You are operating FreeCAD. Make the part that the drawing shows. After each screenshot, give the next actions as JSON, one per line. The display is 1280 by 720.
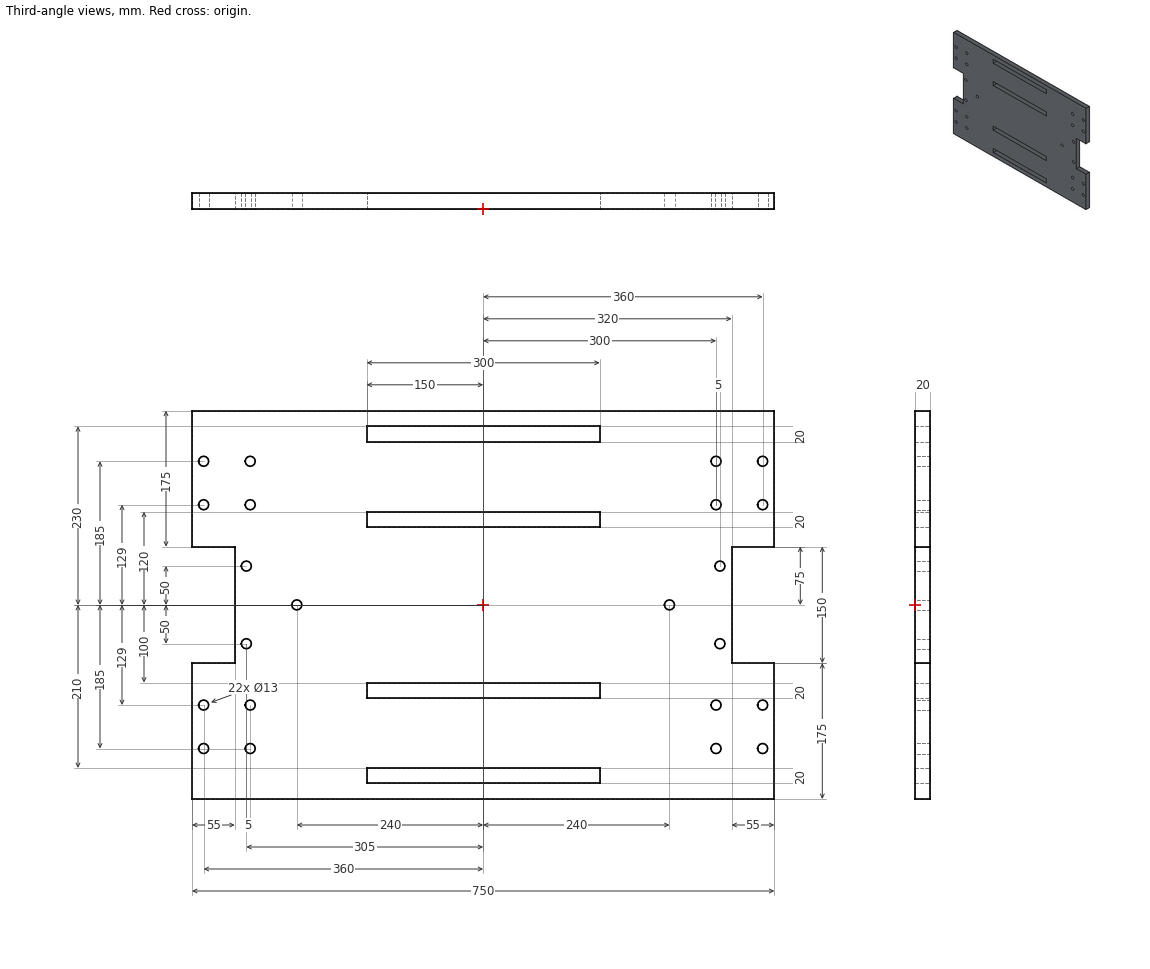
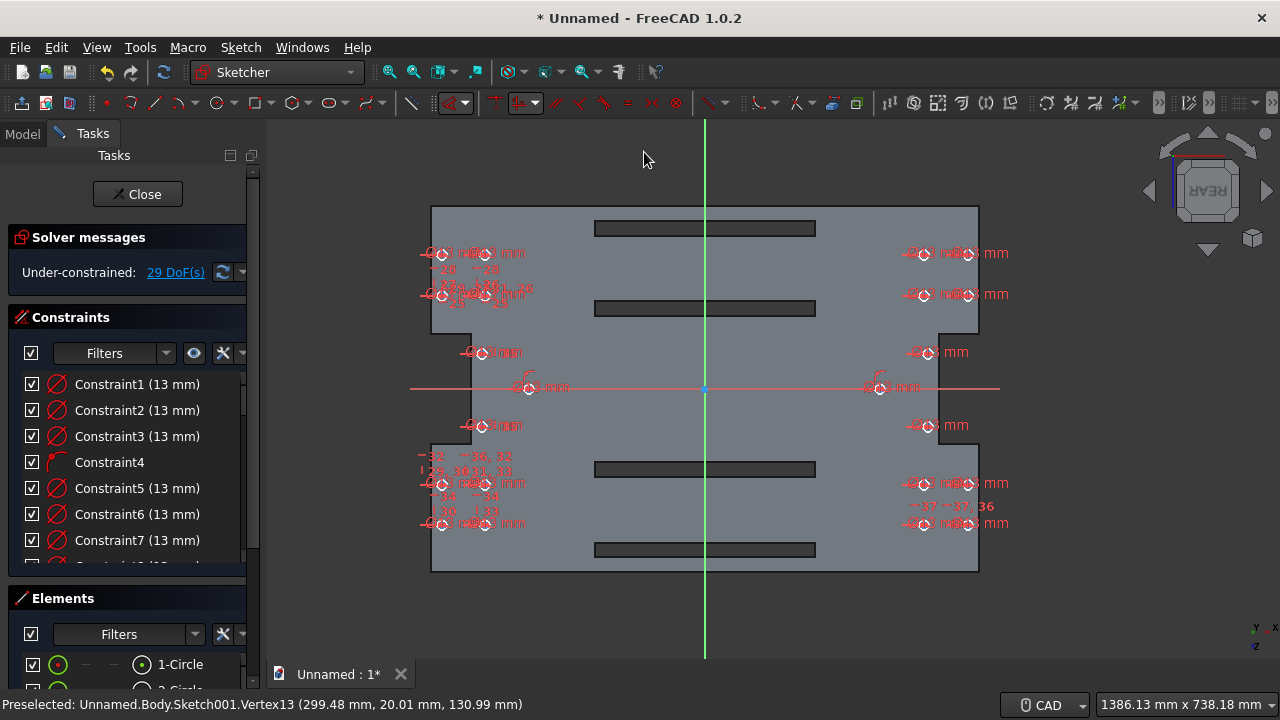
{"action": "left_click", "coordinate": [968, 485]}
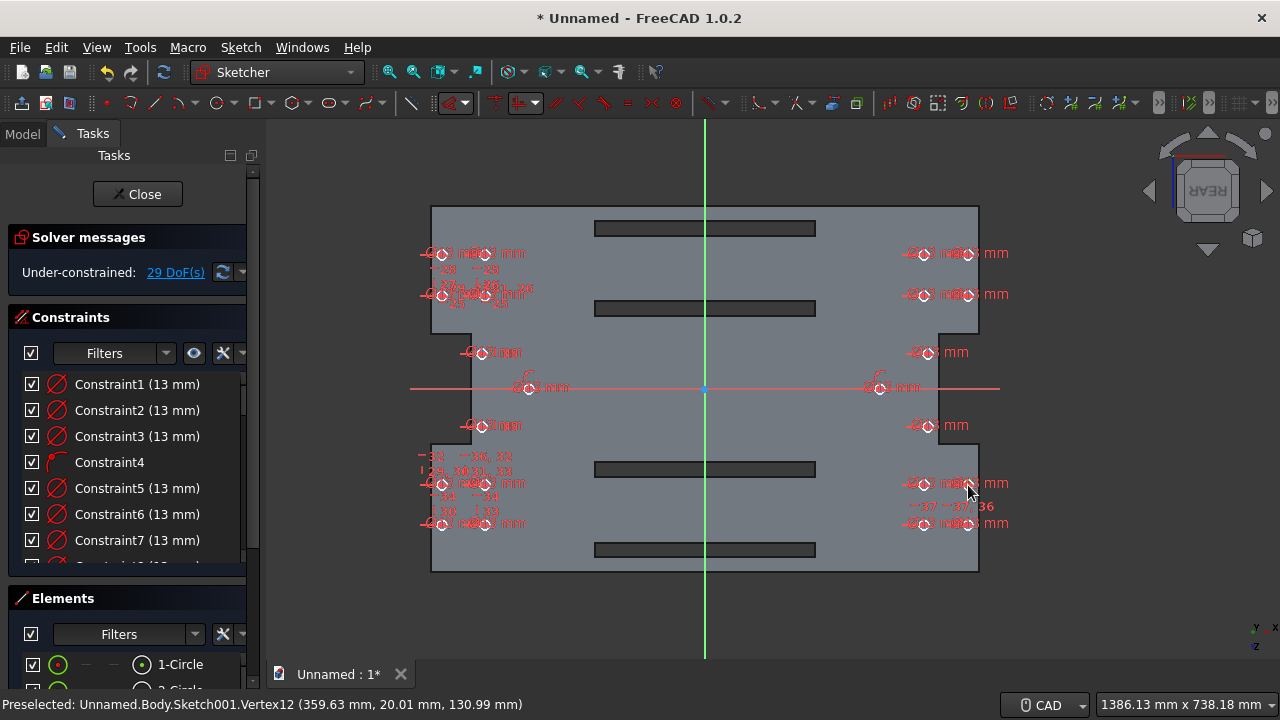
{"action": "left_click", "coordinate": [968, 525]}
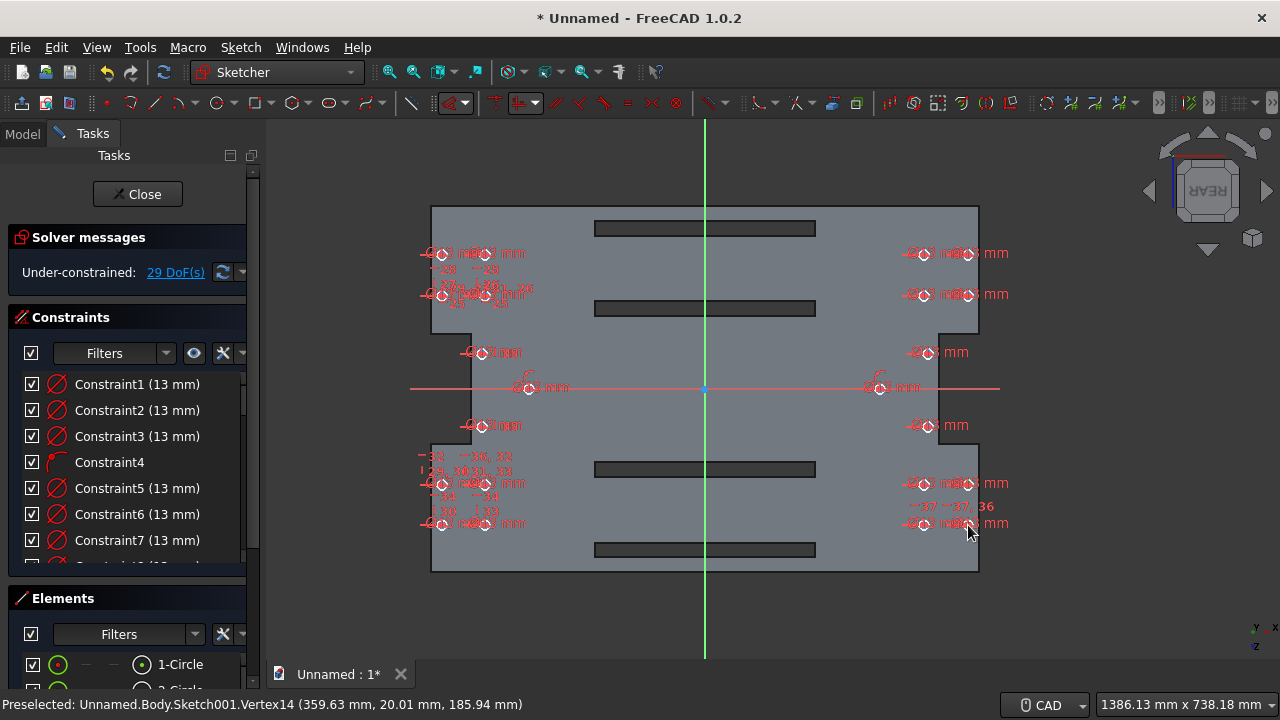
{"action": "left_click", "coordinate": [538, 104]}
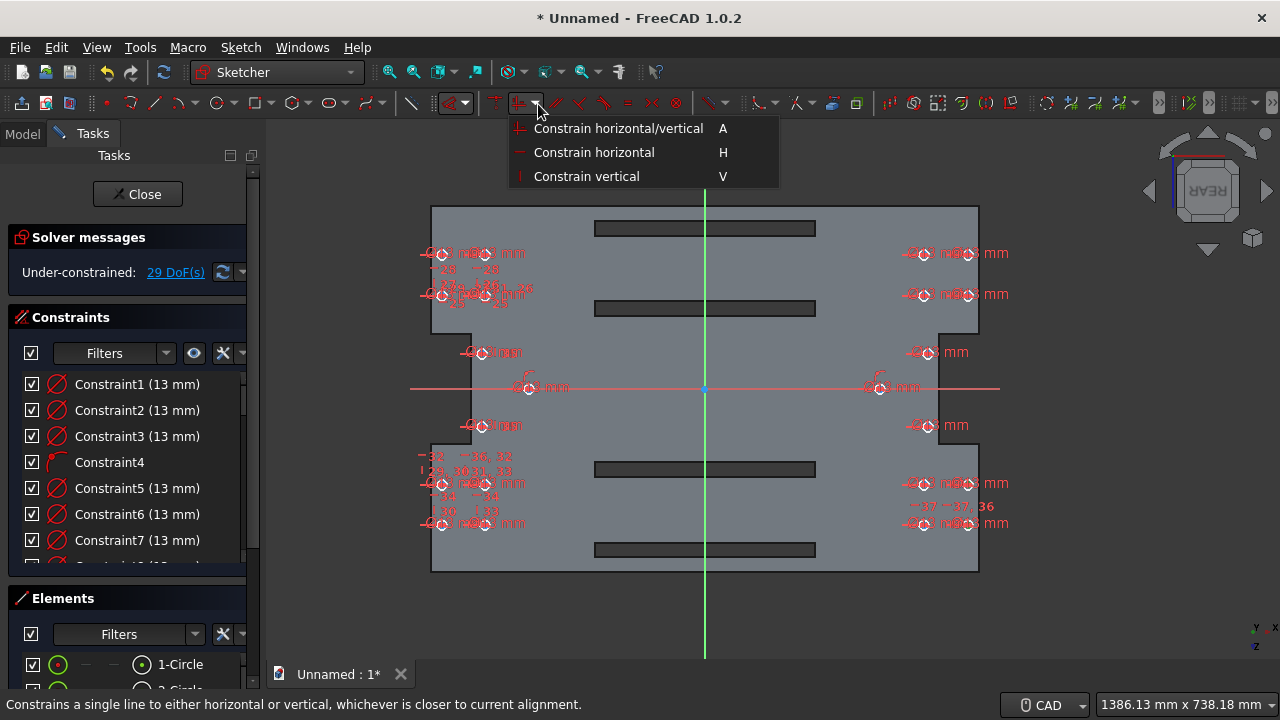
{"action": "left_click", "coordinate": [644, 176]}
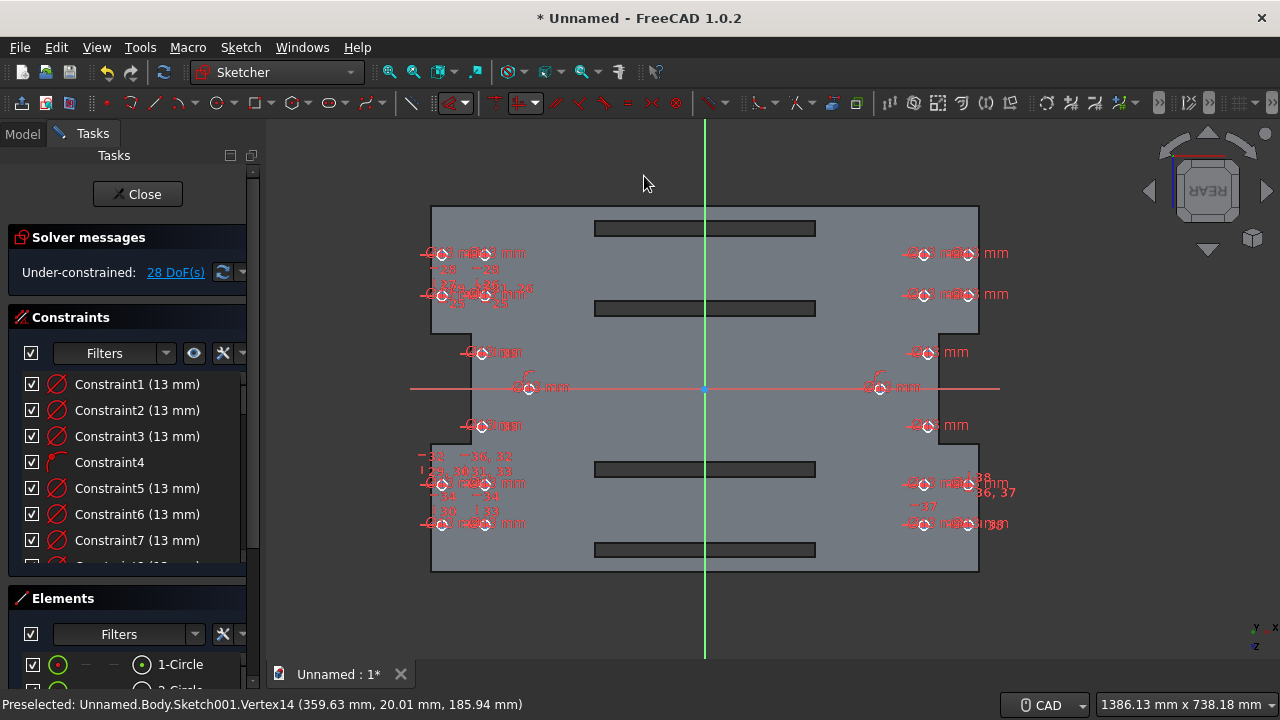
{"action": "left_click", "coordinate": [485, 525]}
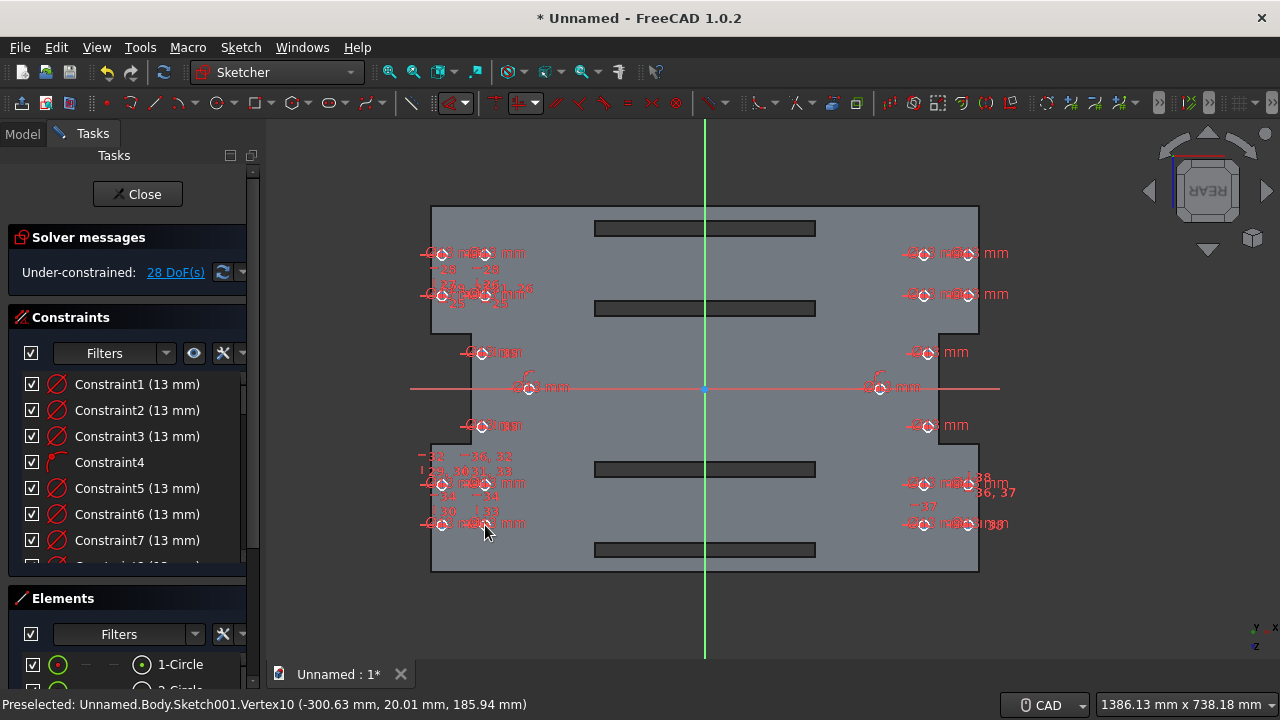
{"action": "left_click", "coordinate": [968, 525]}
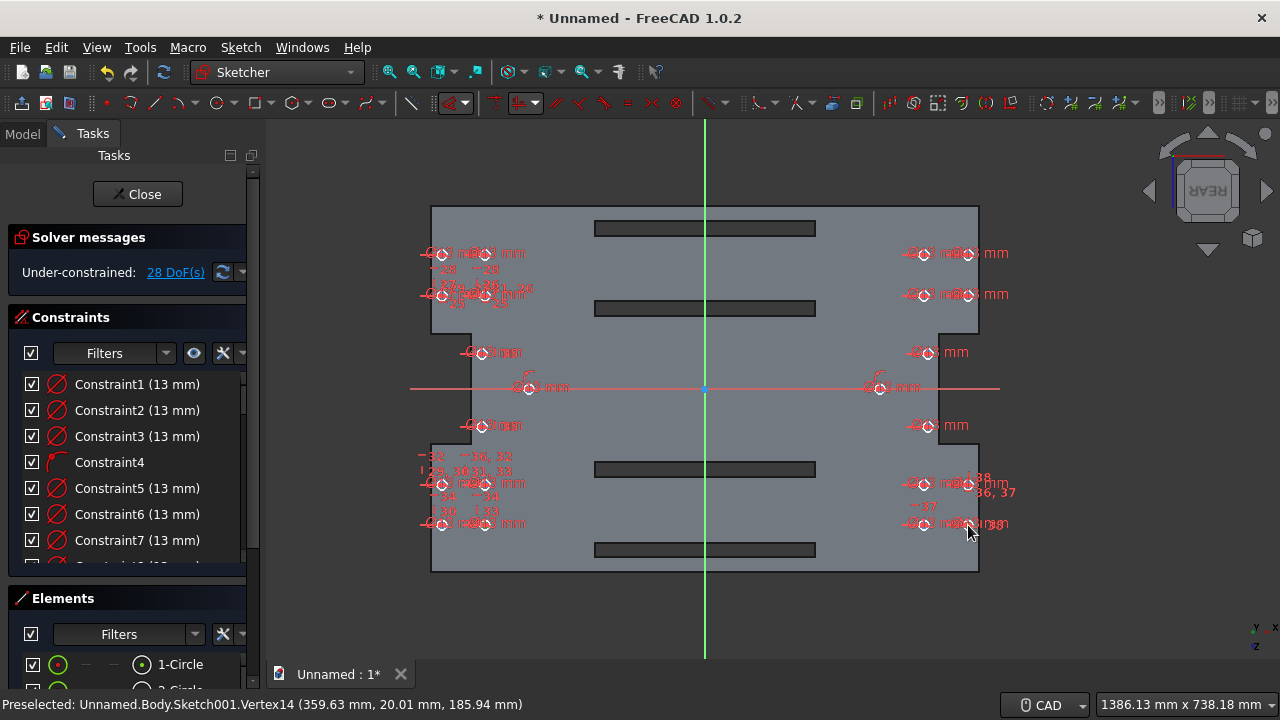
{"action": "left_click", "coordinate": [538, 104]}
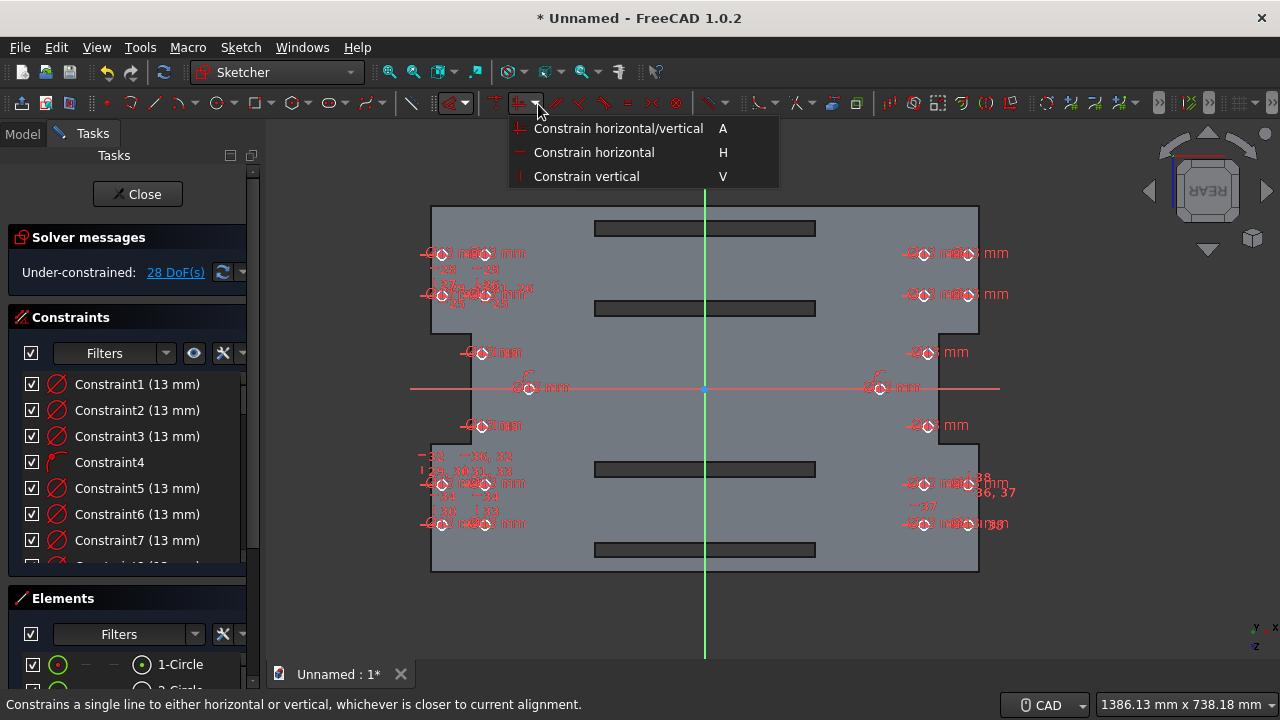
{"action": "left_click", "coordinate": [644, 152]}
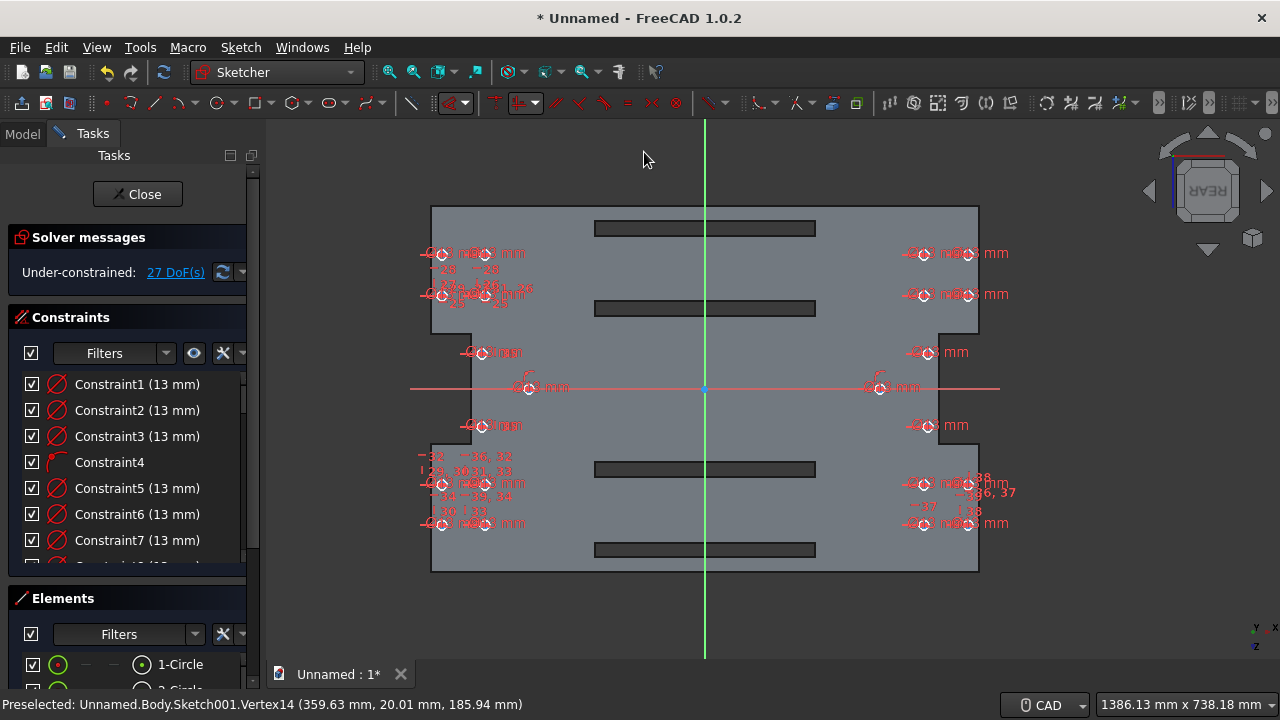
{"action": "left_click", "coordinate": [968, 485]}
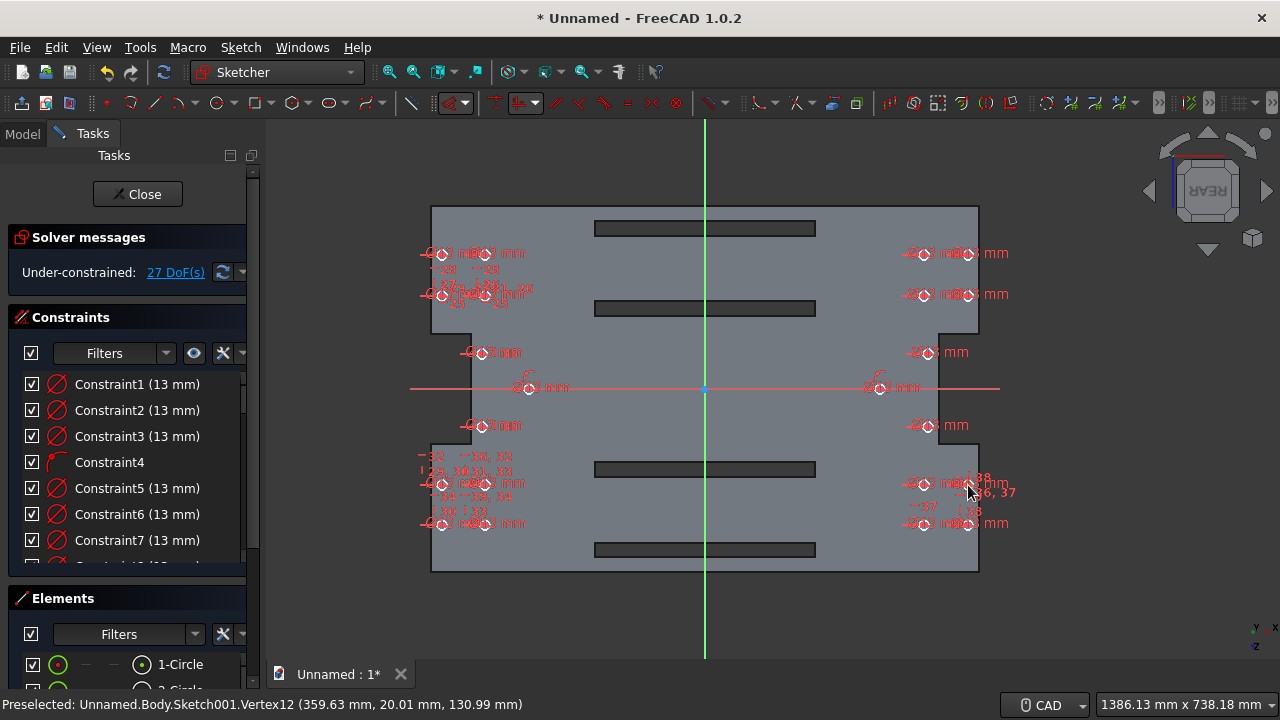
{"action": "left_click", "coordinate": [968, 296]}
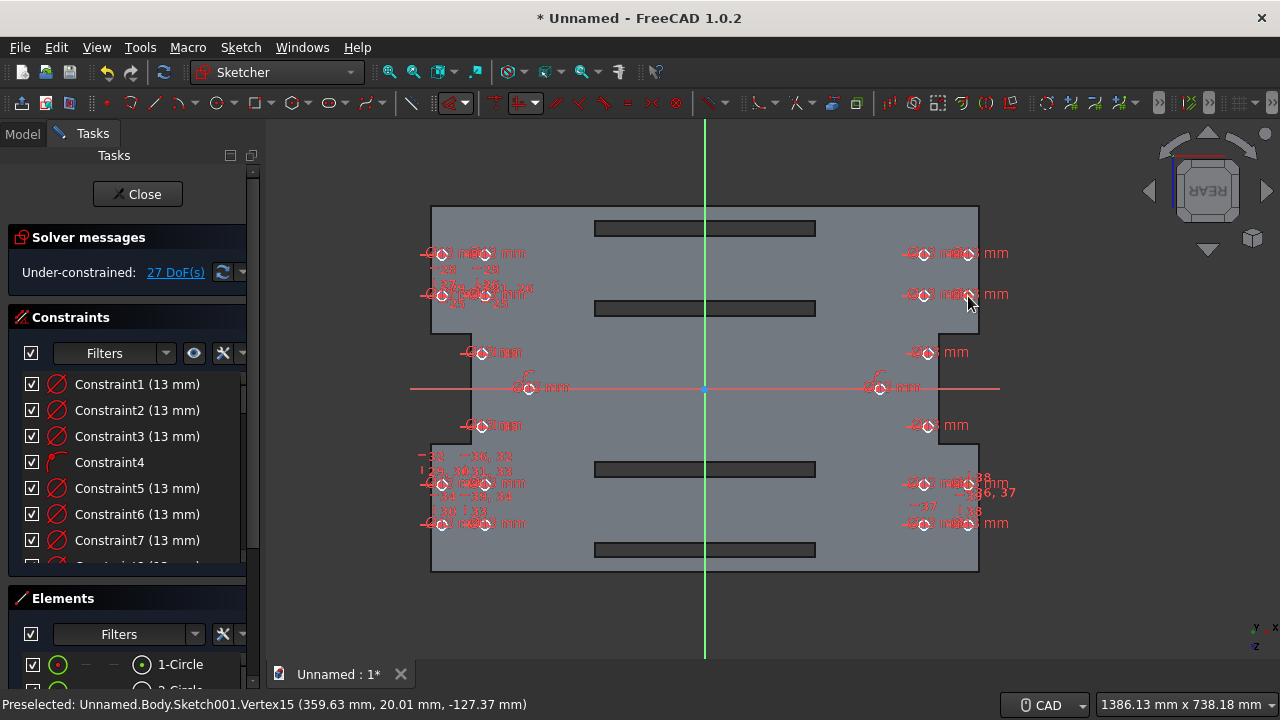
{"action": "left_click", "coordinate": [538, 104]}